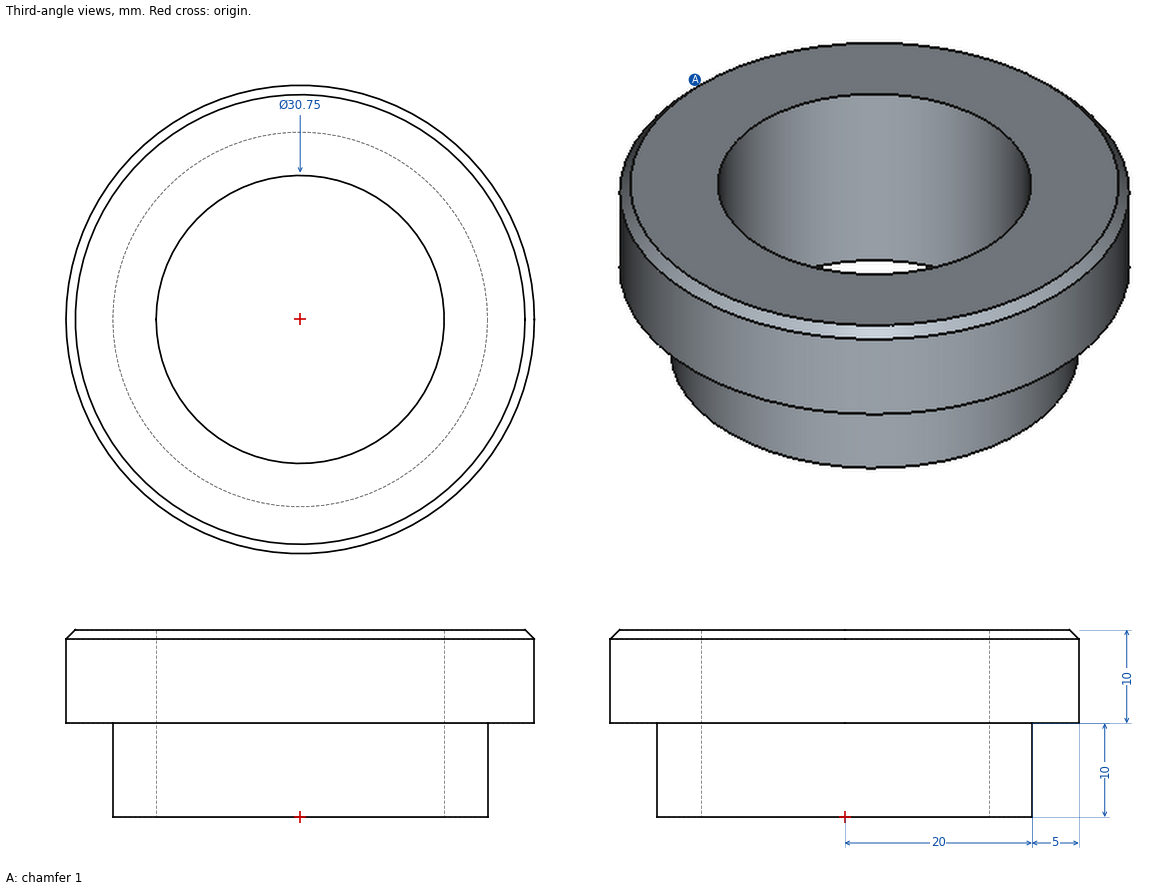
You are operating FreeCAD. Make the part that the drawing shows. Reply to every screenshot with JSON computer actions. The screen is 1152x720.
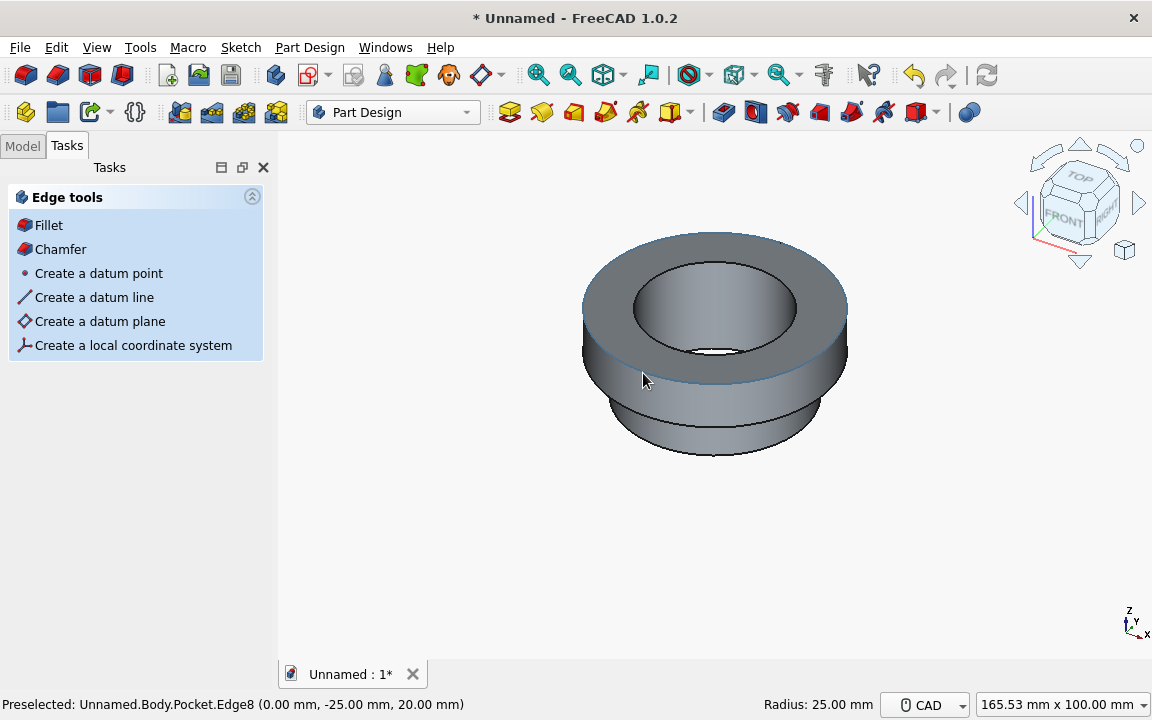
{"action": "left_click", "coordinate": [58, 76]}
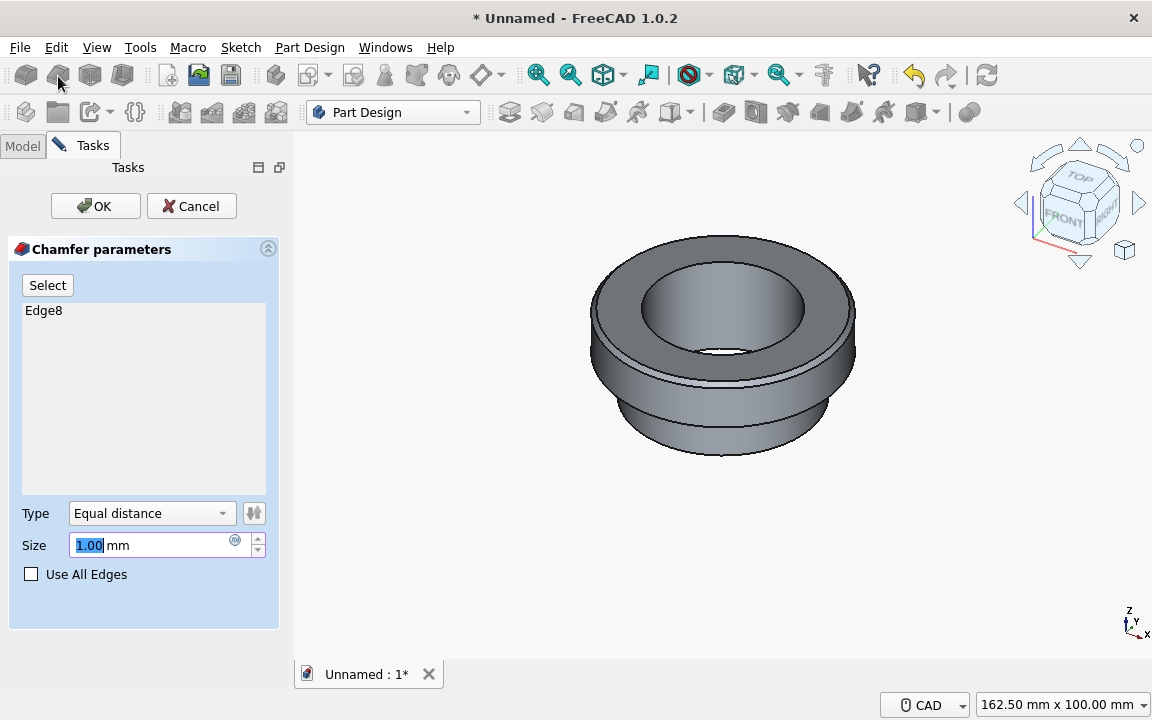
{"action": "type", "text": "1"}
{"action": "key", "text": "Tab"}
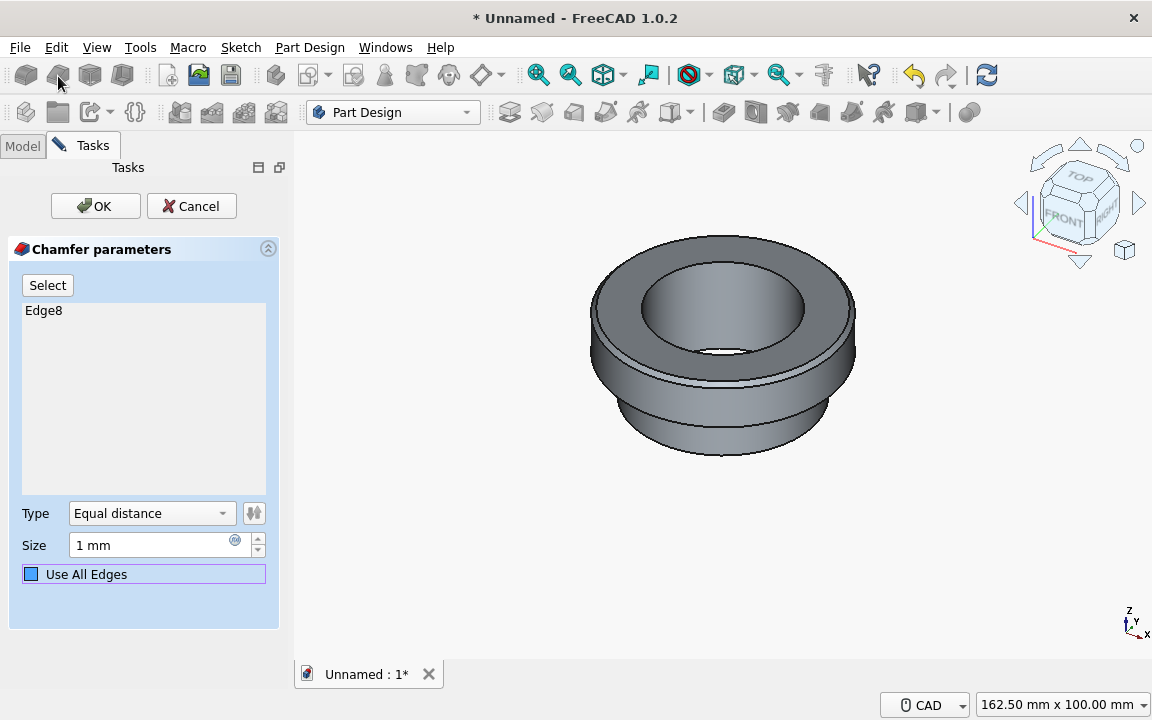
{"action": "left_click", "coordinate": [96, 206]}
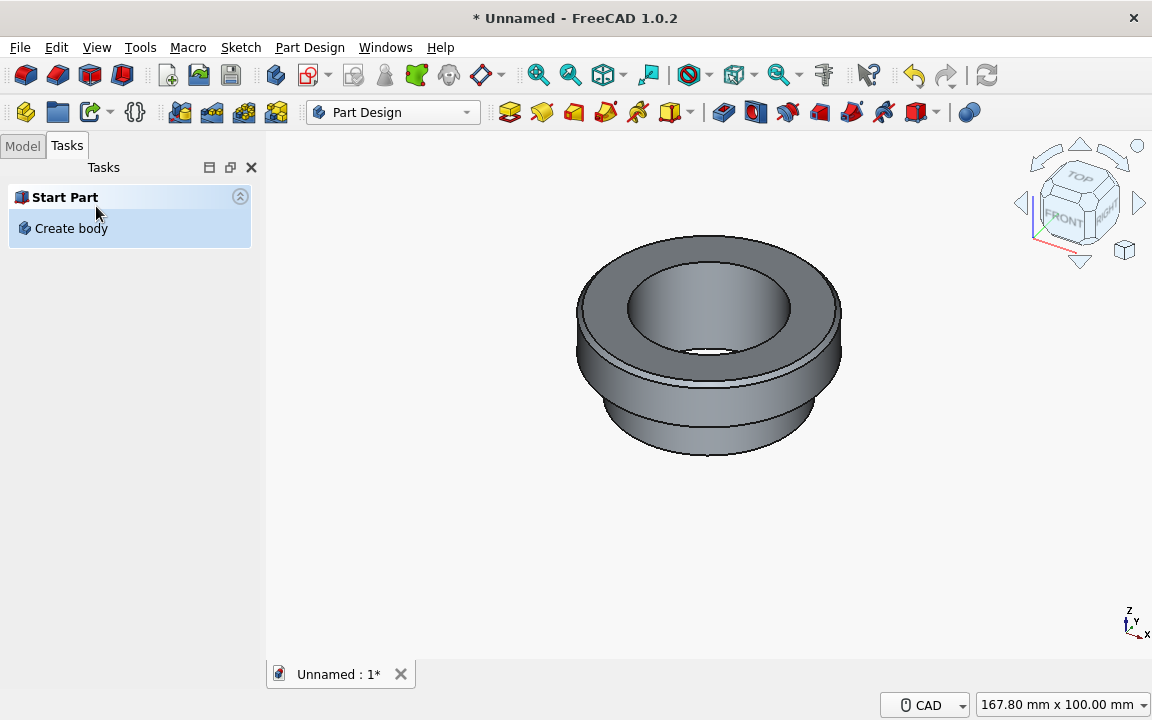
{"action": "key", "text": "0"}